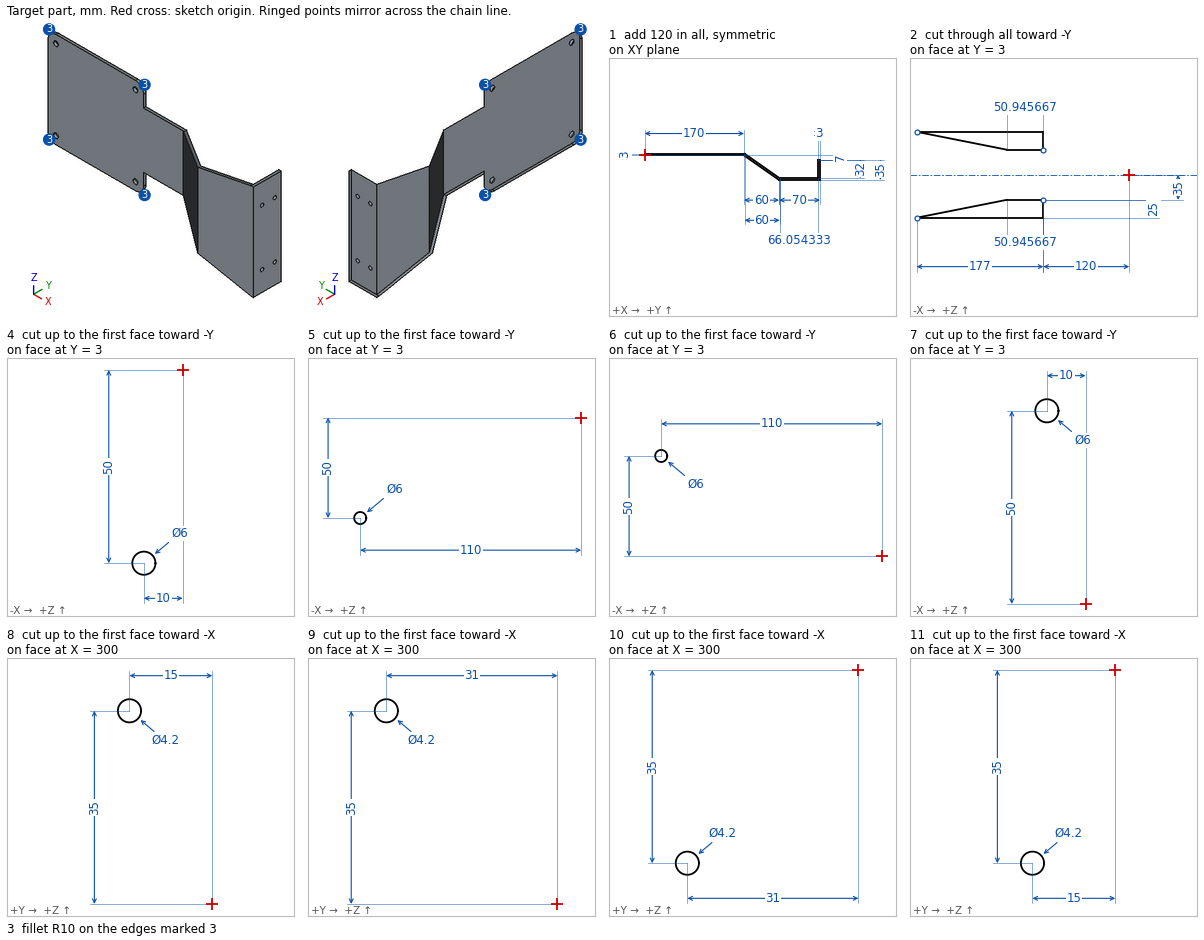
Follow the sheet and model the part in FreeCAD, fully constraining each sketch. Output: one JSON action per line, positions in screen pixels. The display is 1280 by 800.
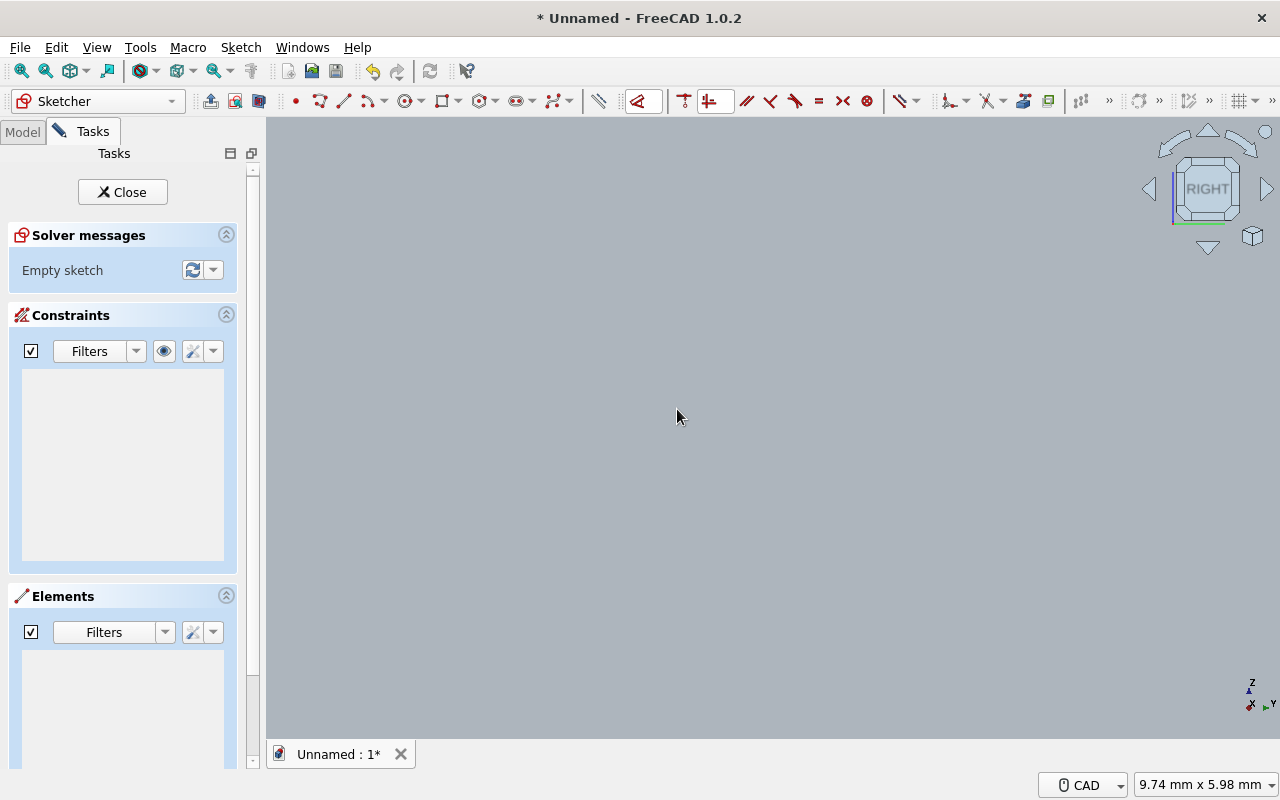
{"action": "left_click", "coordinate": [406, 102]}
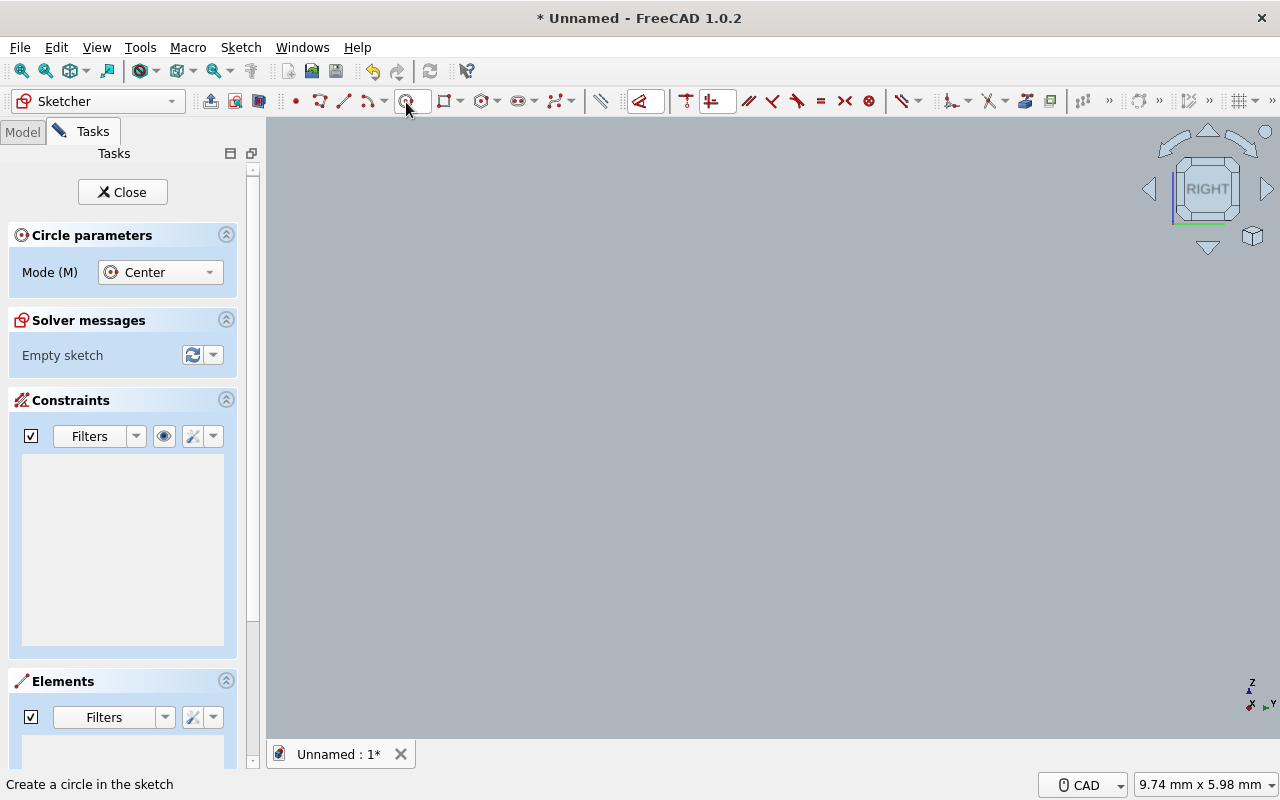
{"action": "left_click", "coordinate": [705, 428]}
{"action": "left_click", "coordinate": [859, 273]}
{"action": "key", "text": "Escape"}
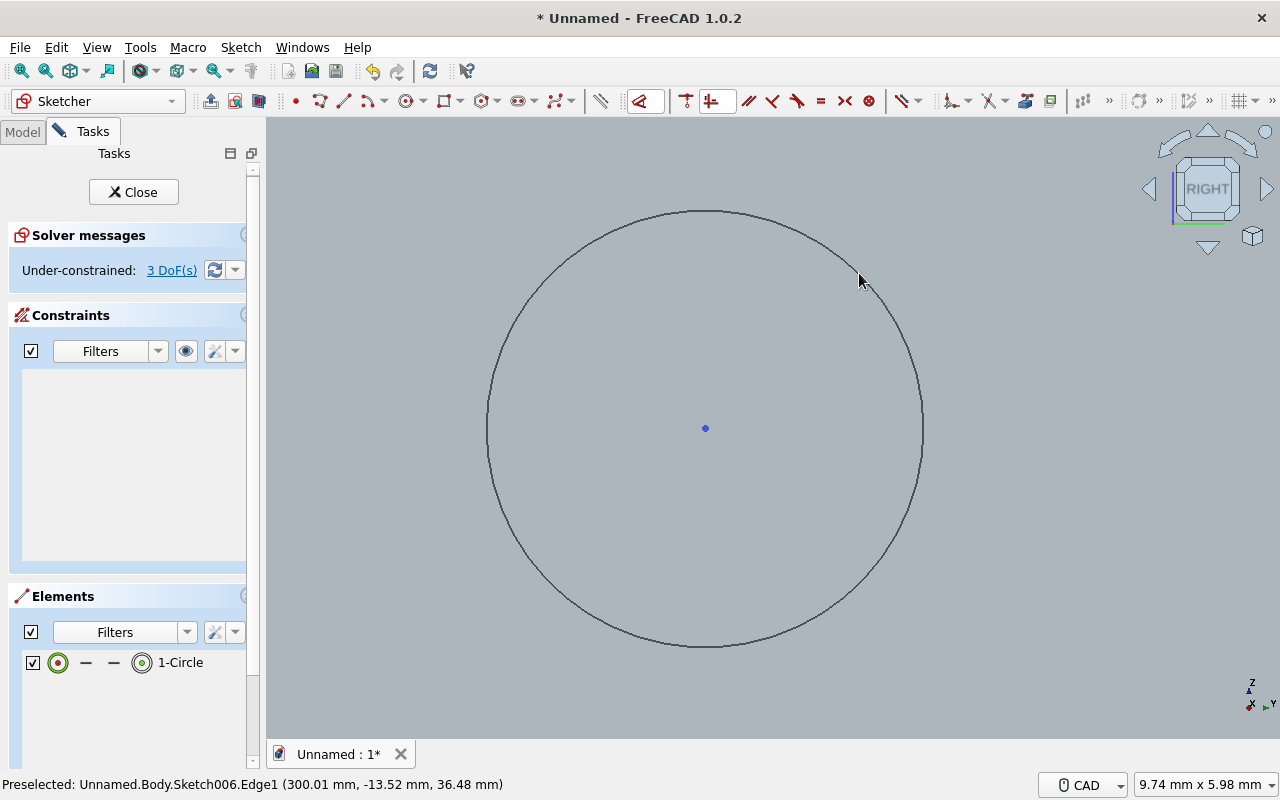
{"action": "left_click", "coordinate": [859, 274]}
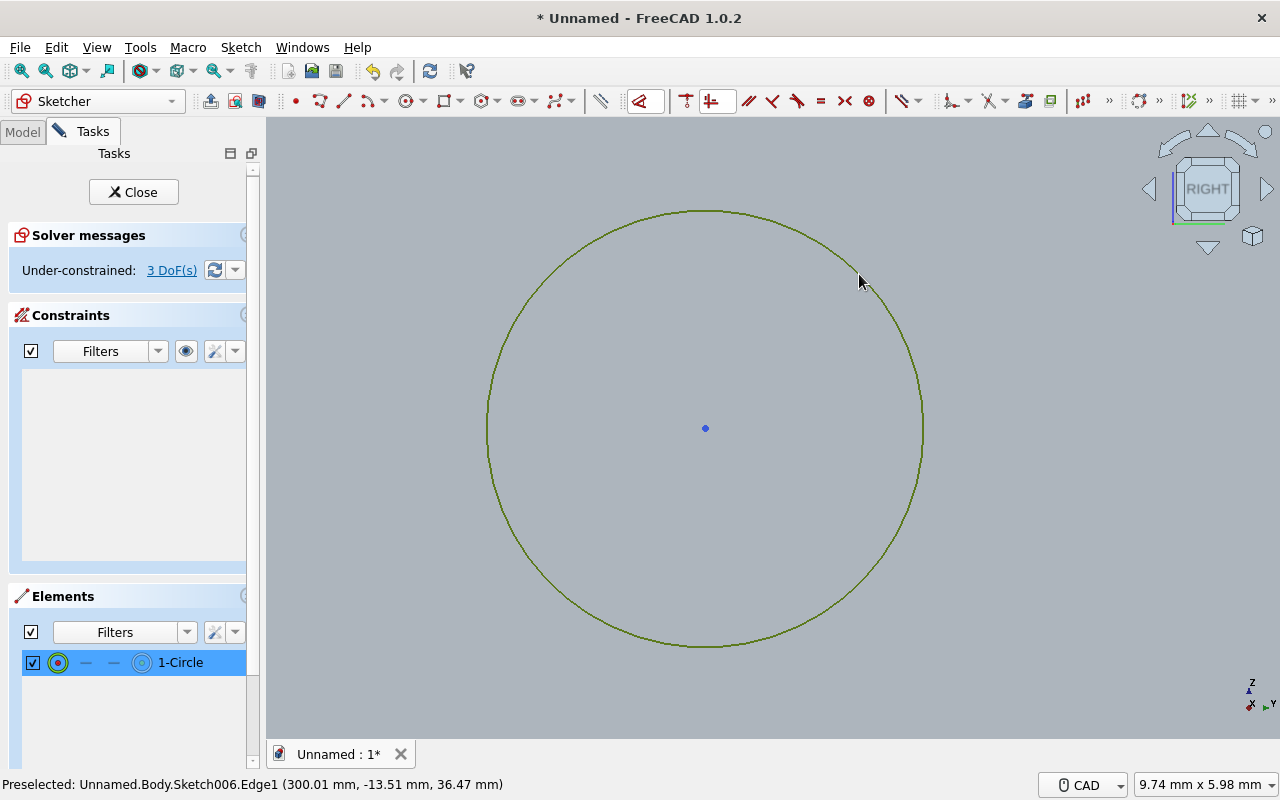
{"action": "left_click", "coordinate": [658, 102]}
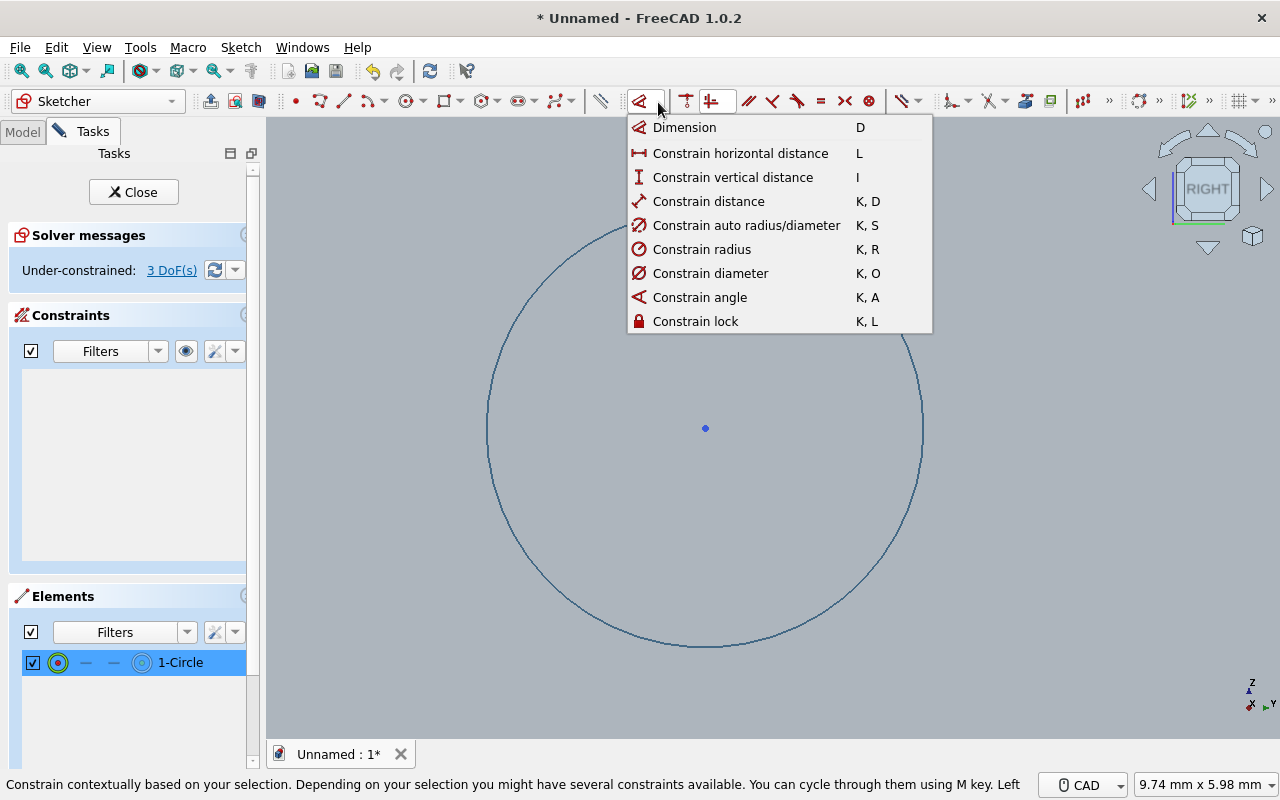
{"action": "left_click", "coordinate": [780, 273]}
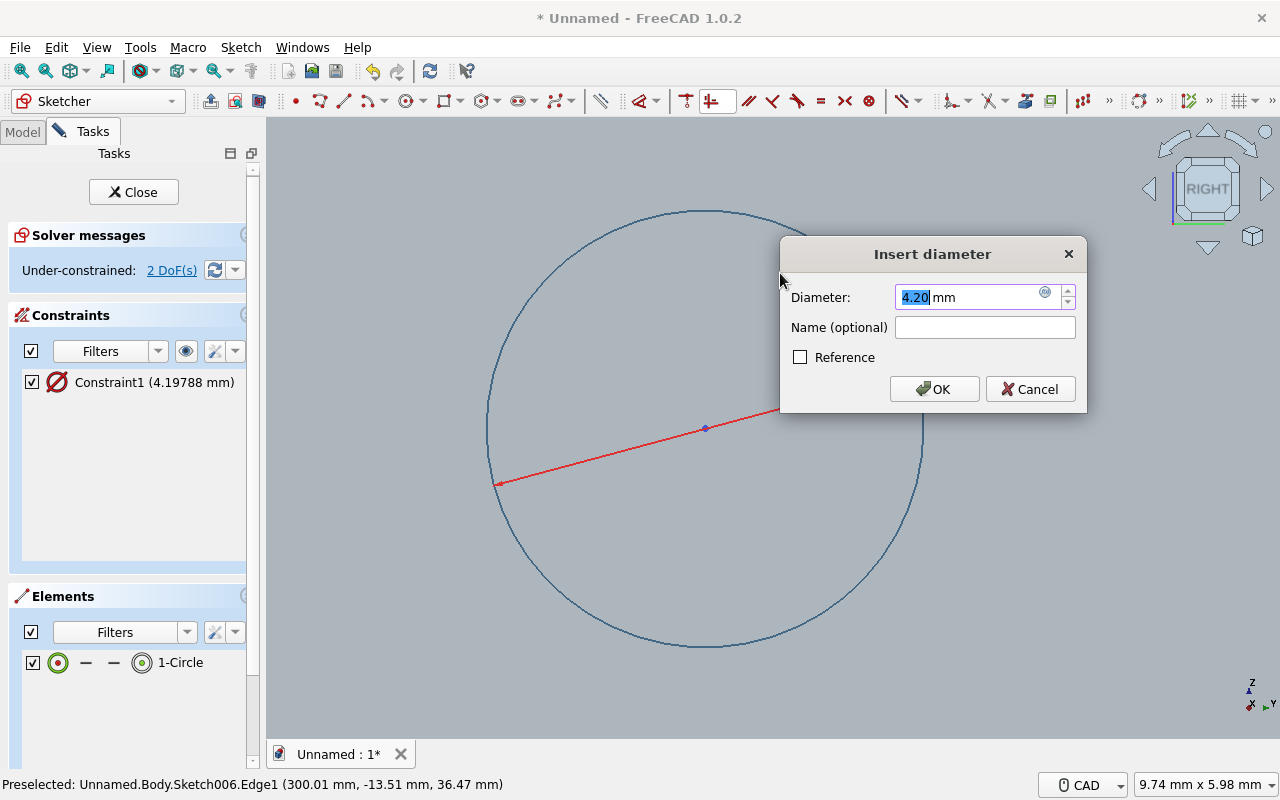
{"action": "type", "text": "4.2"}
{"action": "key", "text": "Return"}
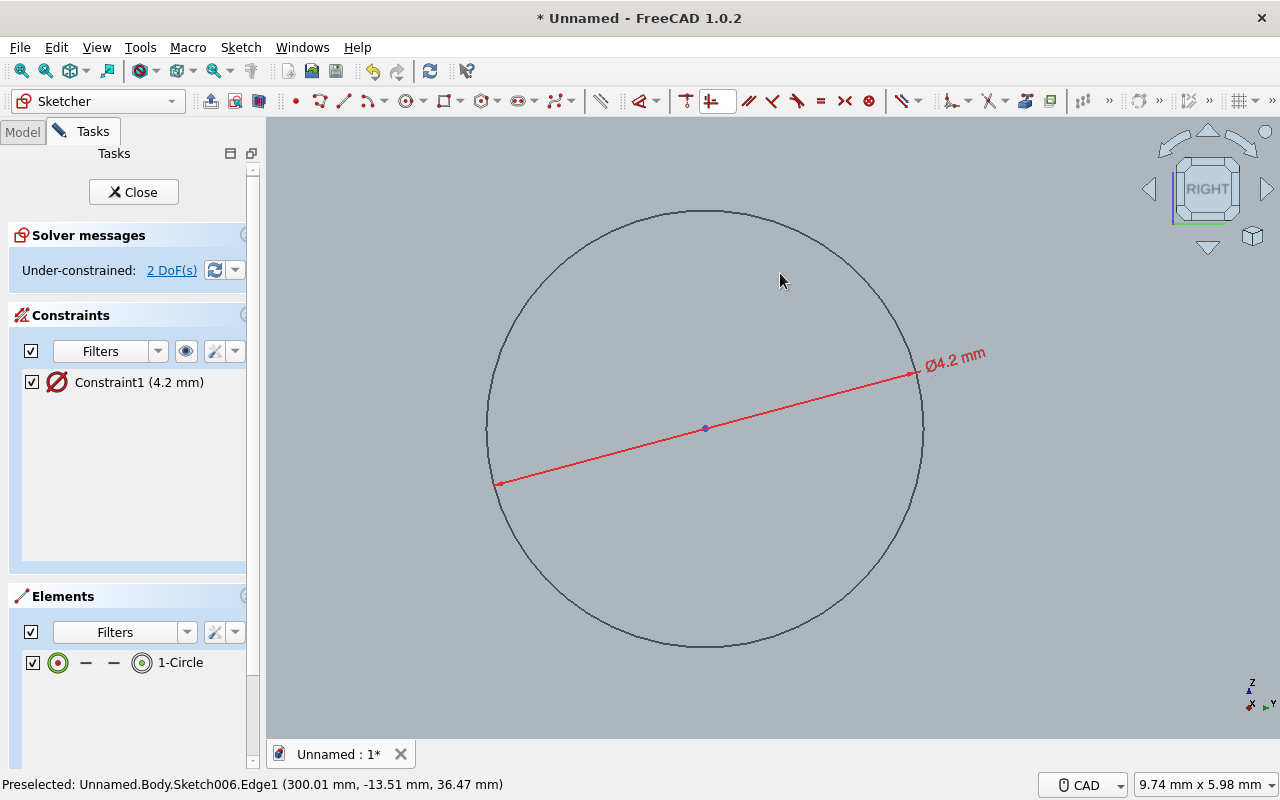
{"action": "left_click", "coordinate": [705, 429]}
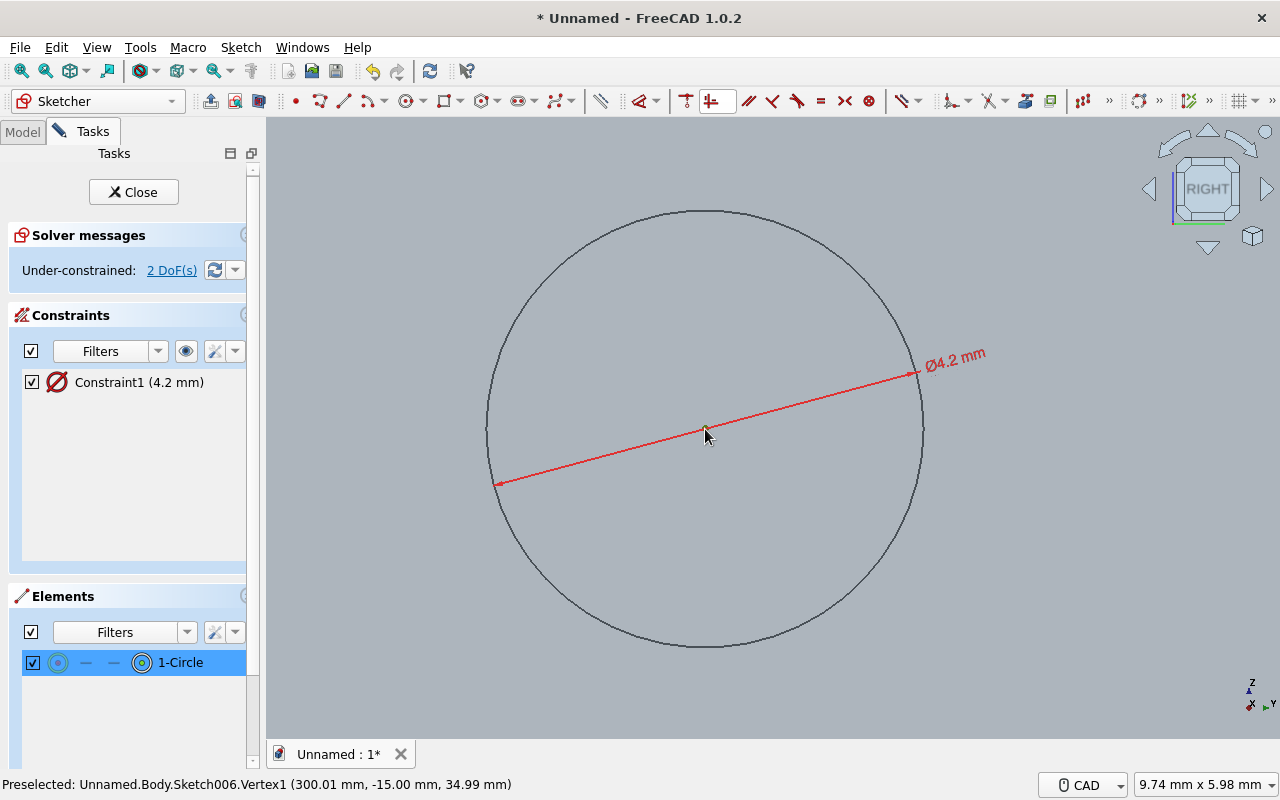
{"action": "left_click", "coordinate": [658, 102]}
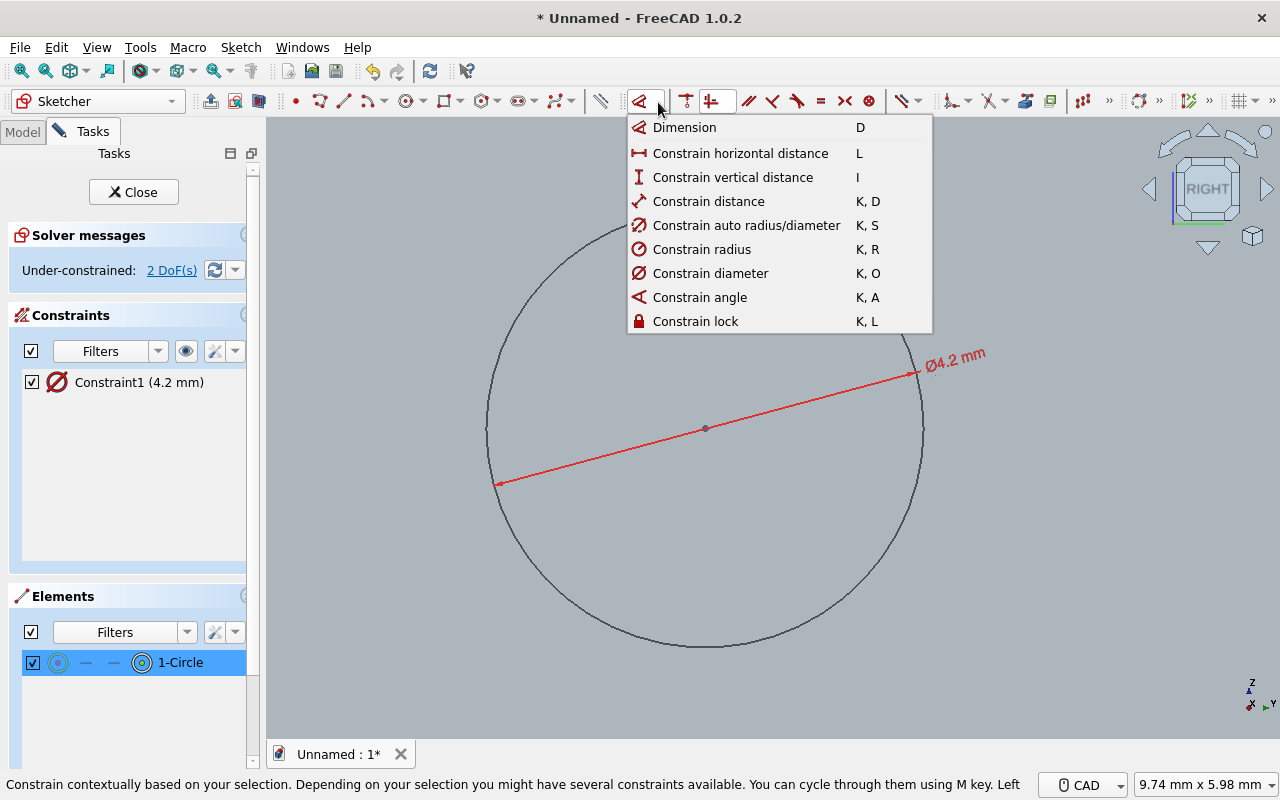
{"action": "left_click", "coordinate": [780, 153]}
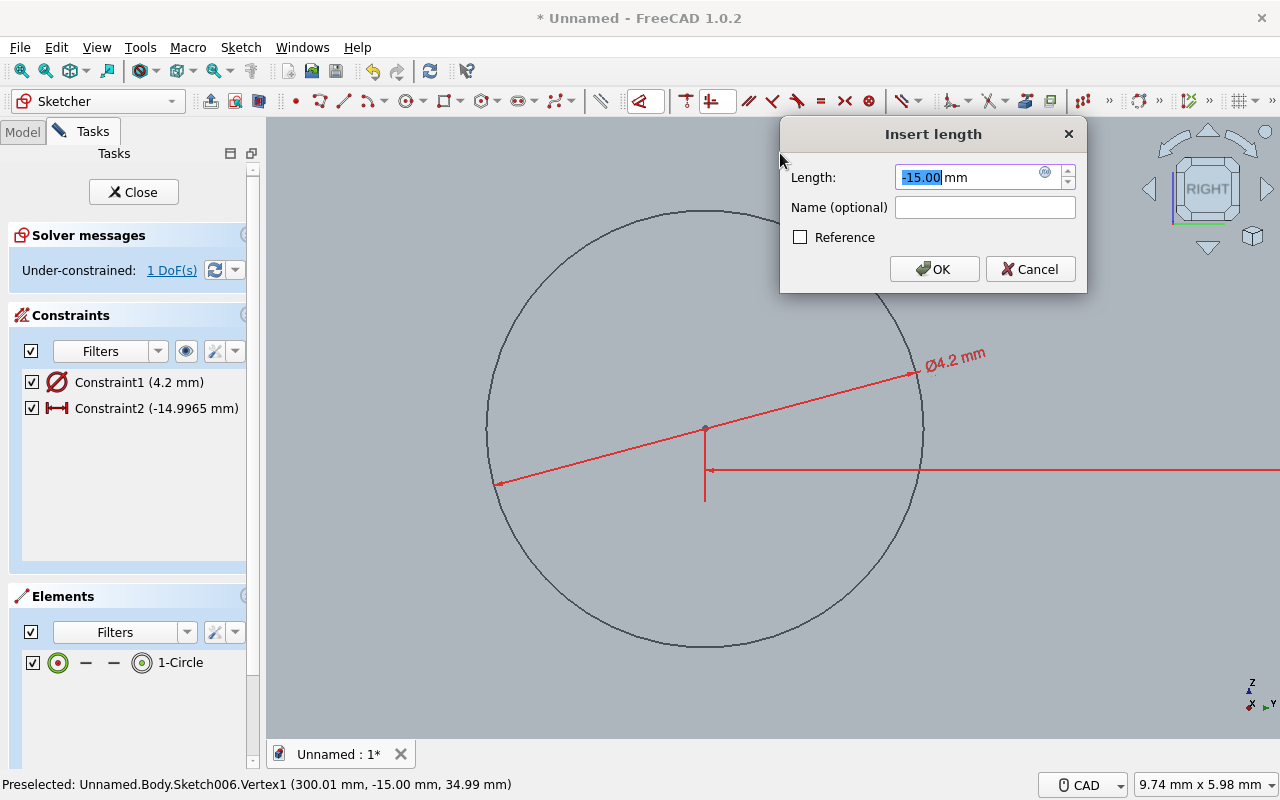
{"action": "type", "text": "-15"}
{"action": "key", "text": "Return"}